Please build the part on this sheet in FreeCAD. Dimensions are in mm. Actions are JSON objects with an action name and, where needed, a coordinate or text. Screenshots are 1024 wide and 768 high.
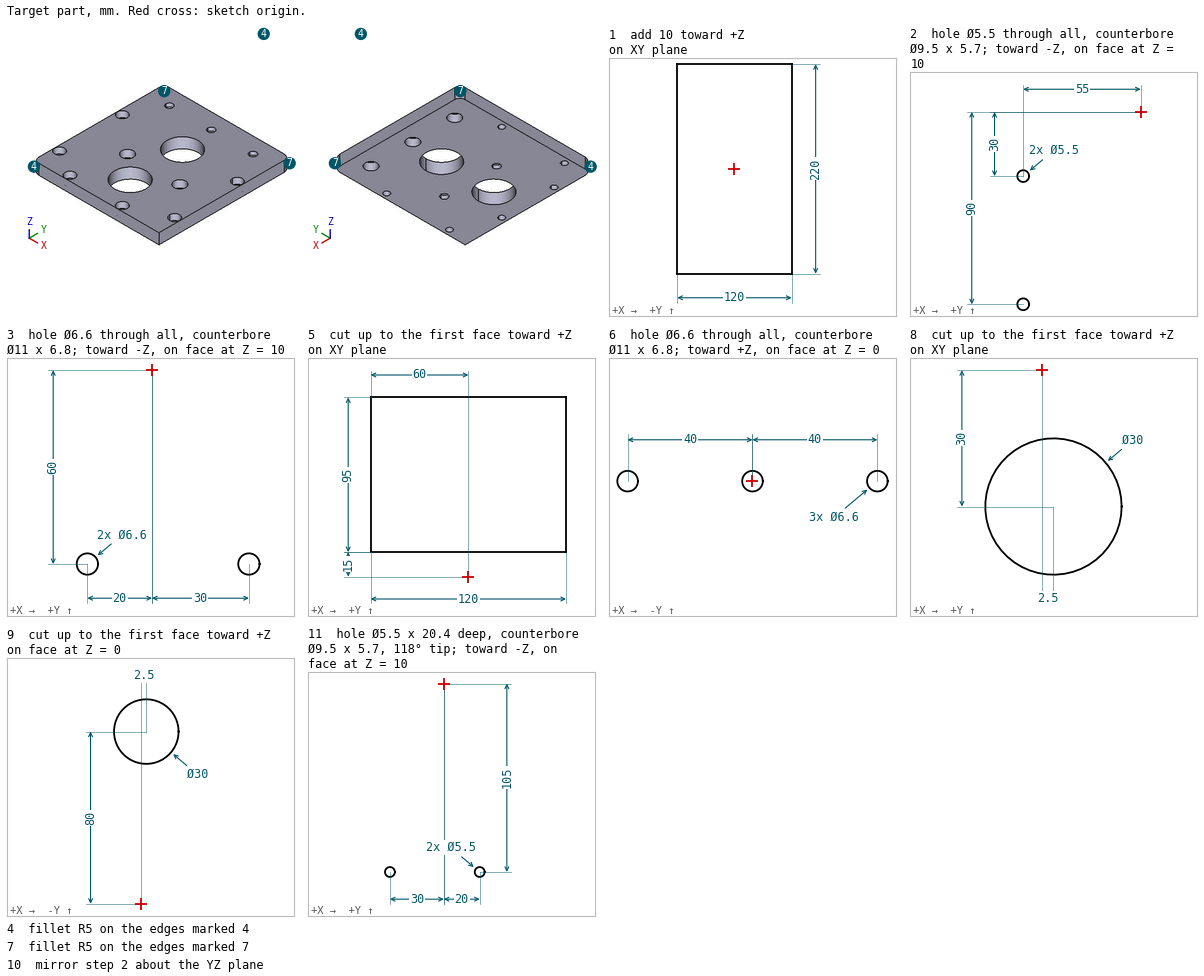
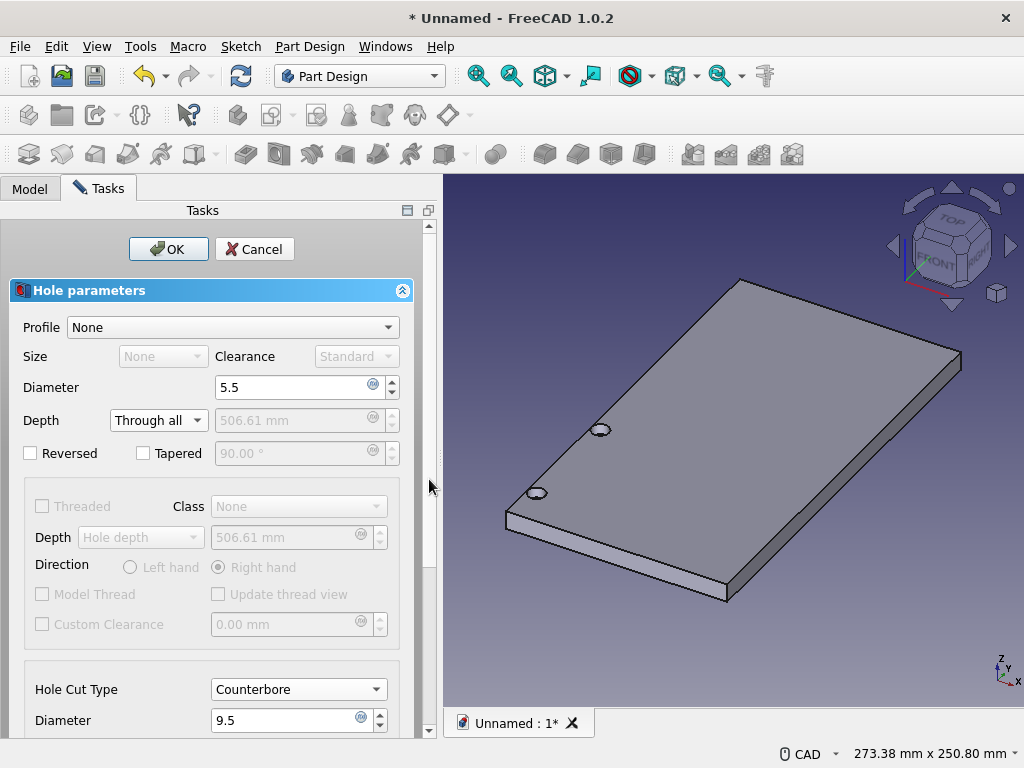
{"action": "left_click", "coordinate": [169, 249]}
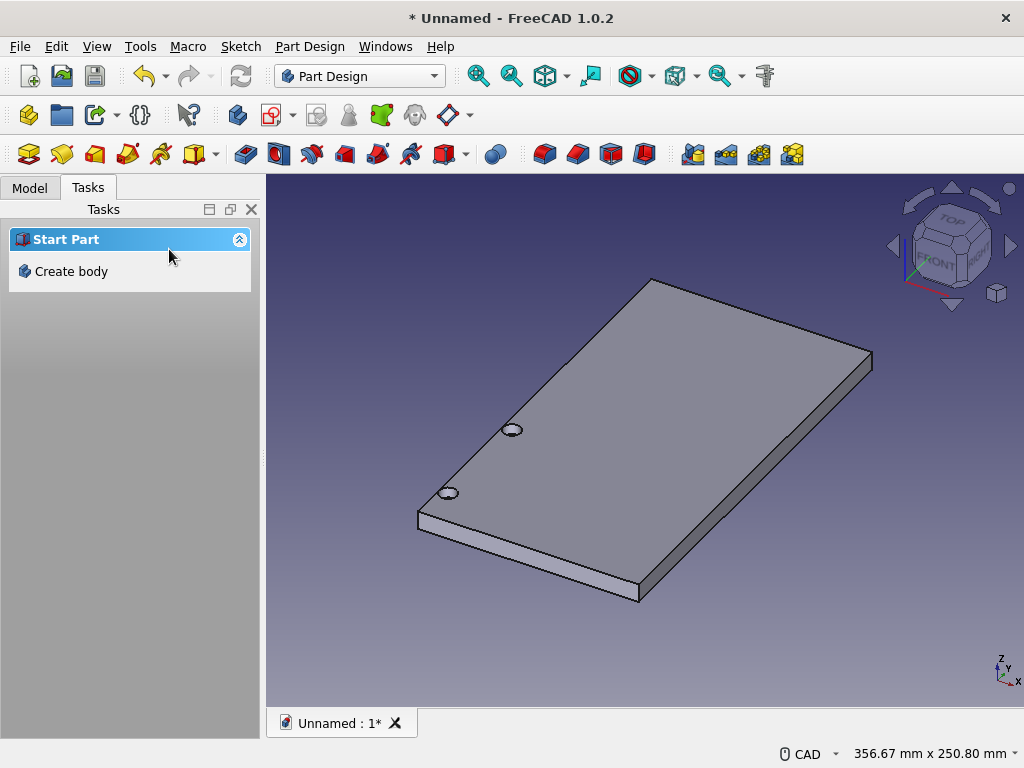
{"action": "left_click", "coordinate": [678, 398]}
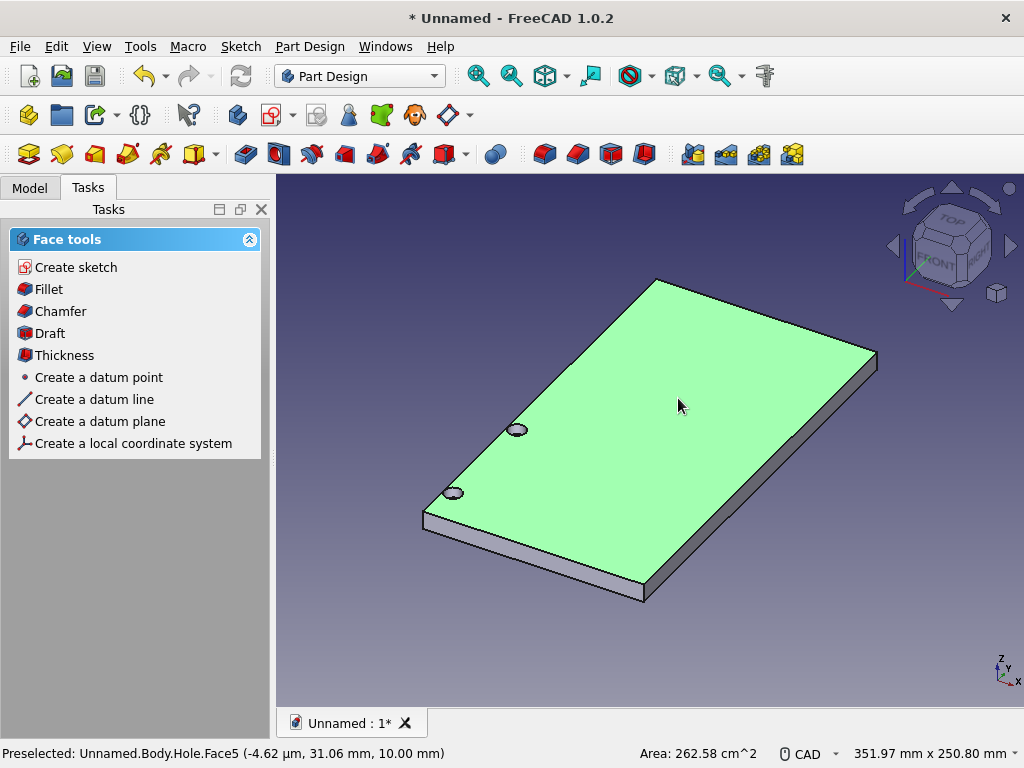
{"action": "left_click", "coordinate": [270, 116]}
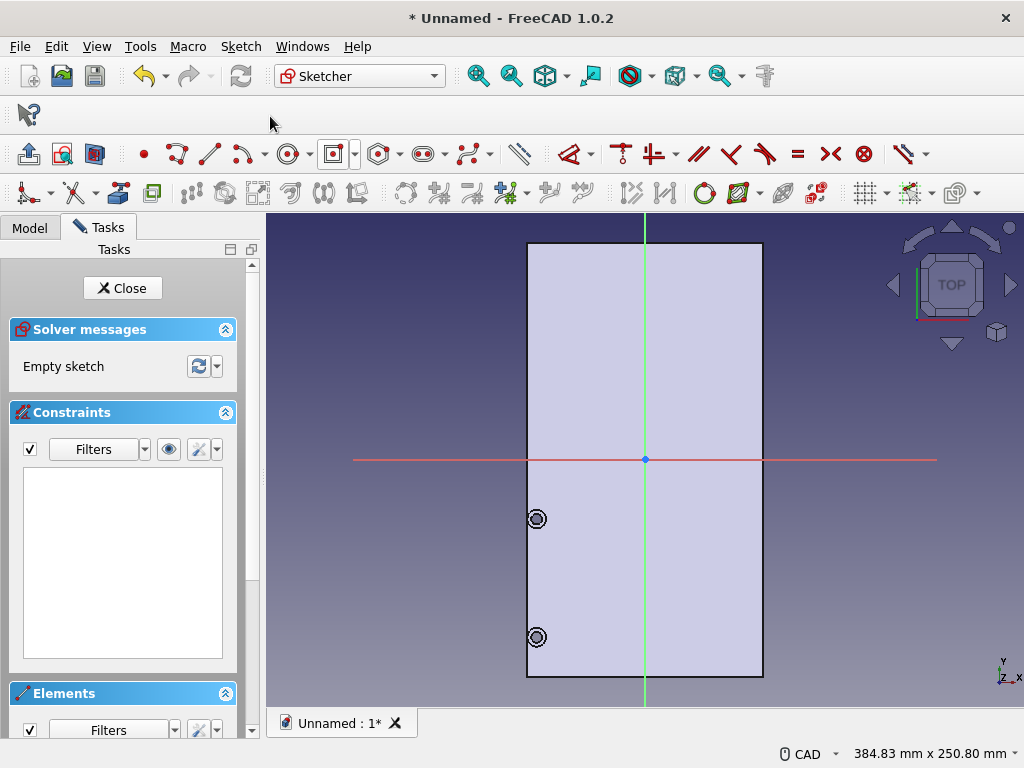
{"action": "scroll", "coordinate": [700, 559], "scroll_direction": "up", "scroll_amount": 5}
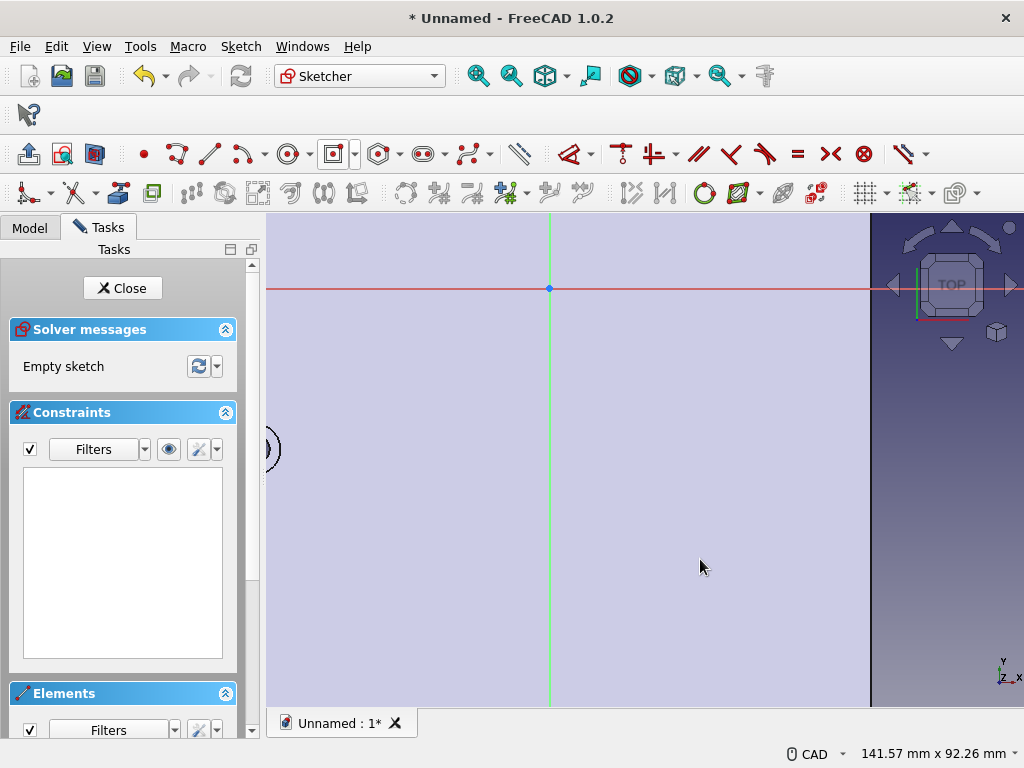
{"action": "left_click", "coordinate": [288, 154]}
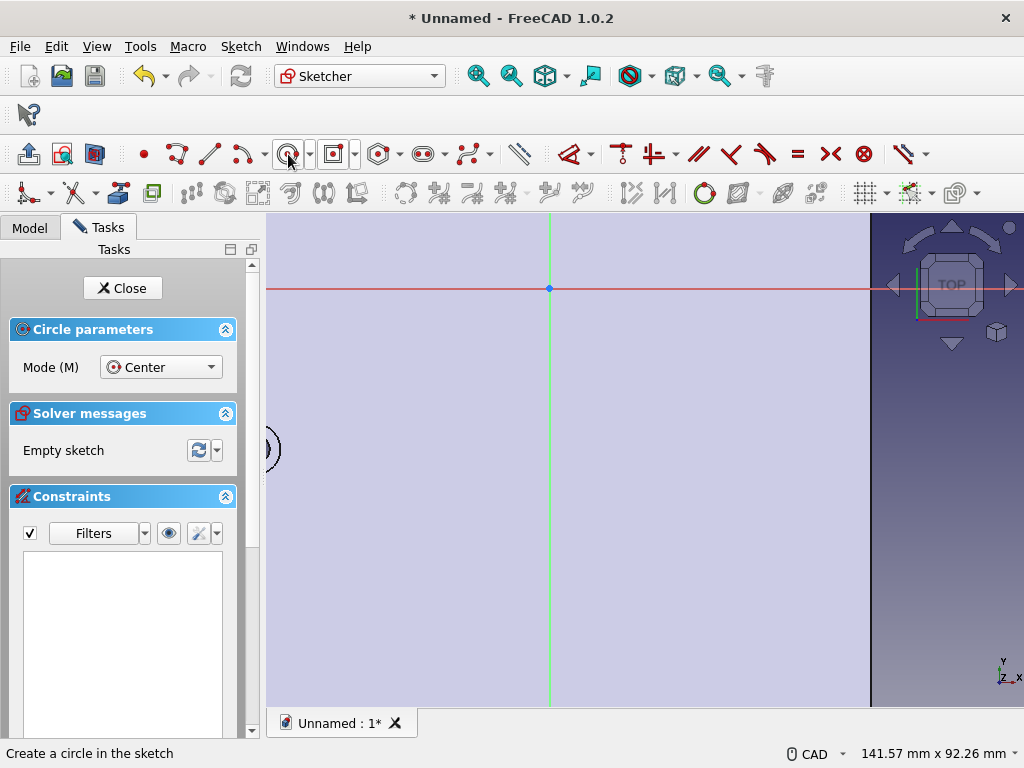
{"action": "scroll", "coordinate": [442, 610], "scroll_direction": "up", "scroll_amount": 2}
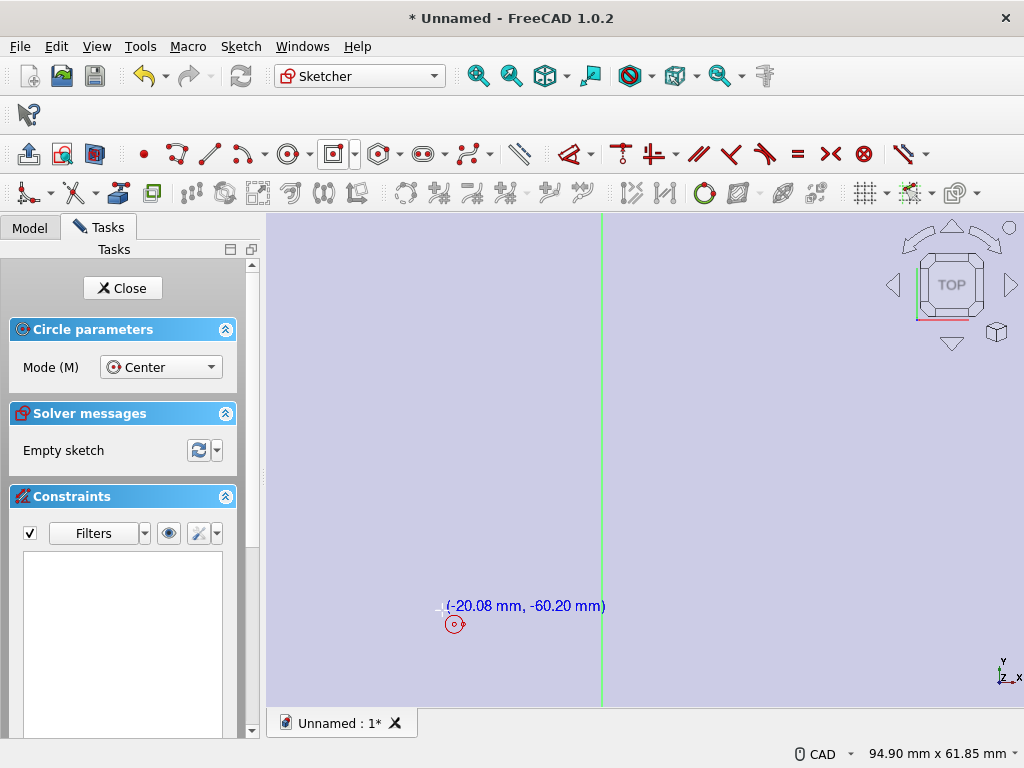
{"action": "left_click", "coordinate": [443, 610]}
{"action": "left_click", "coordinate": [461, 591]}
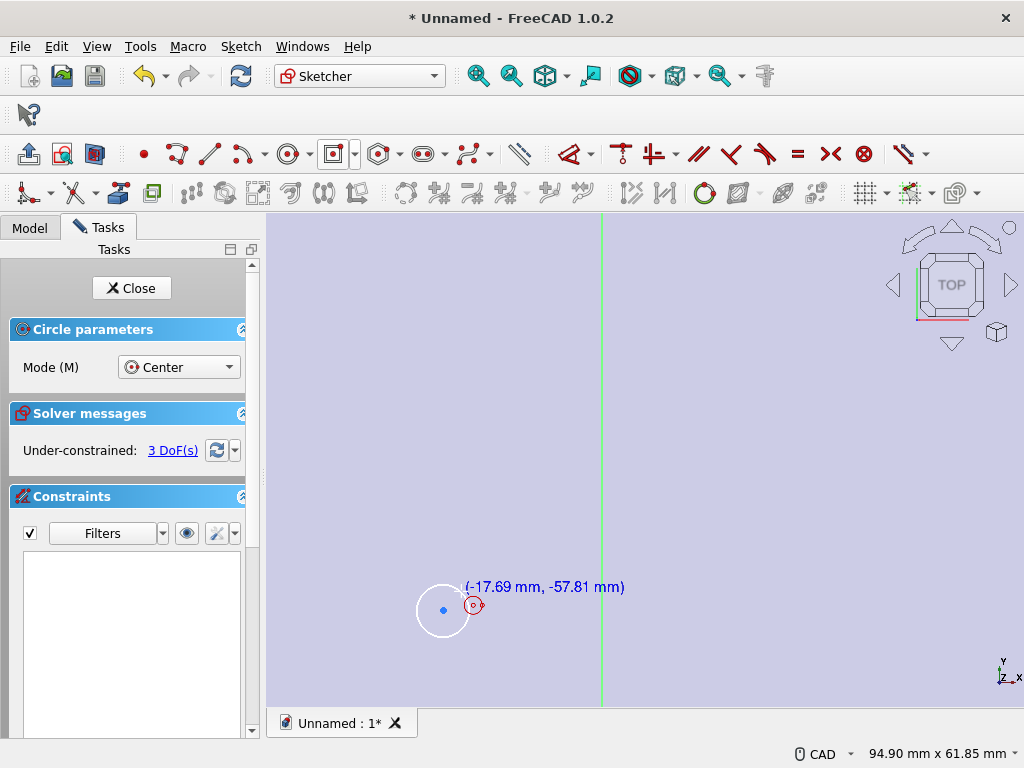
{"action": "left_click", "coordinate": [842, 610]}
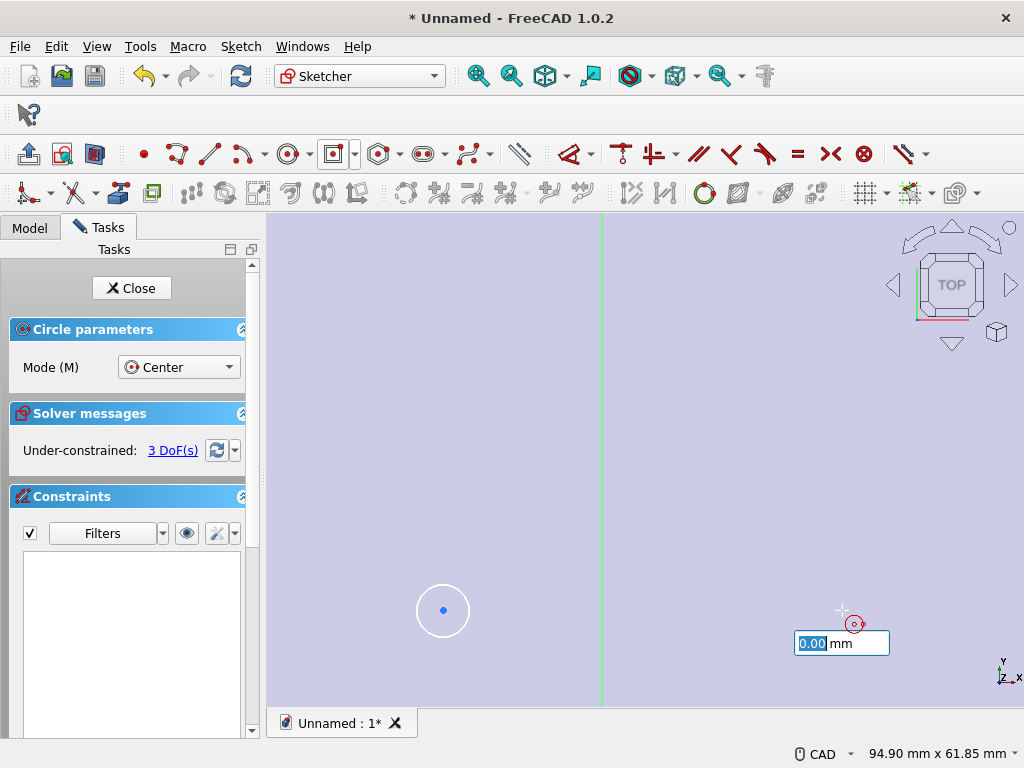
{"action": "scroll", "coordinate": [443, 616], "scroll_direction": "down", "scroll_amount": 2}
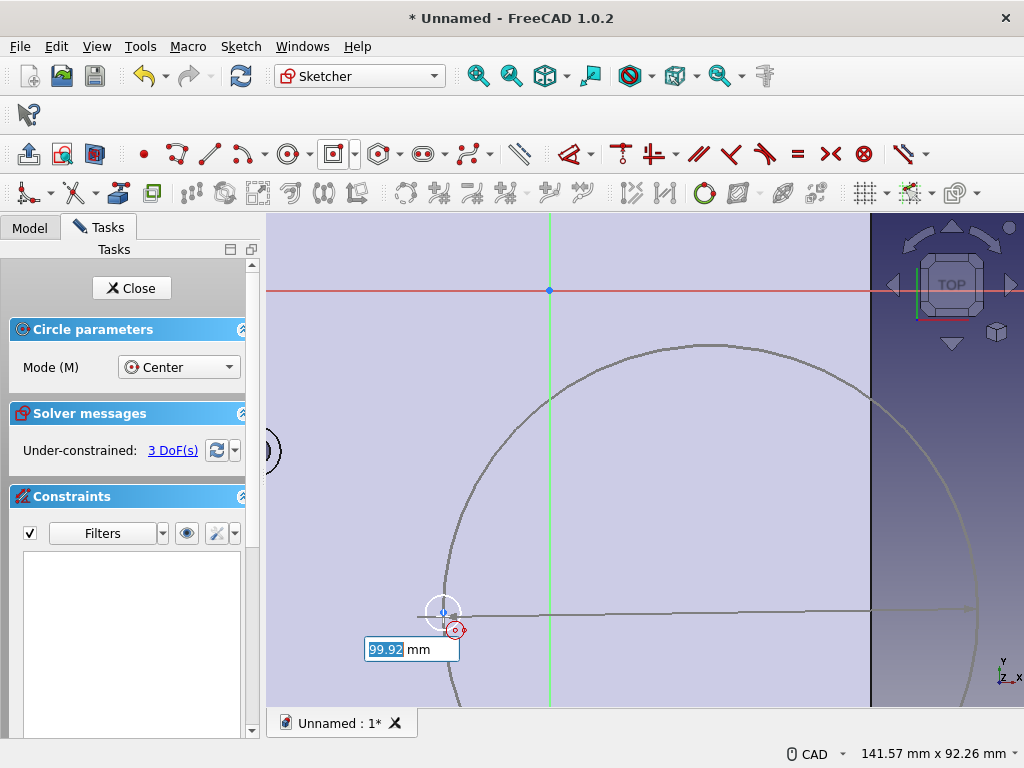
{"action": "left_click", "coordinate": [723, 599]}
{"action": "key", "text": "Escape"}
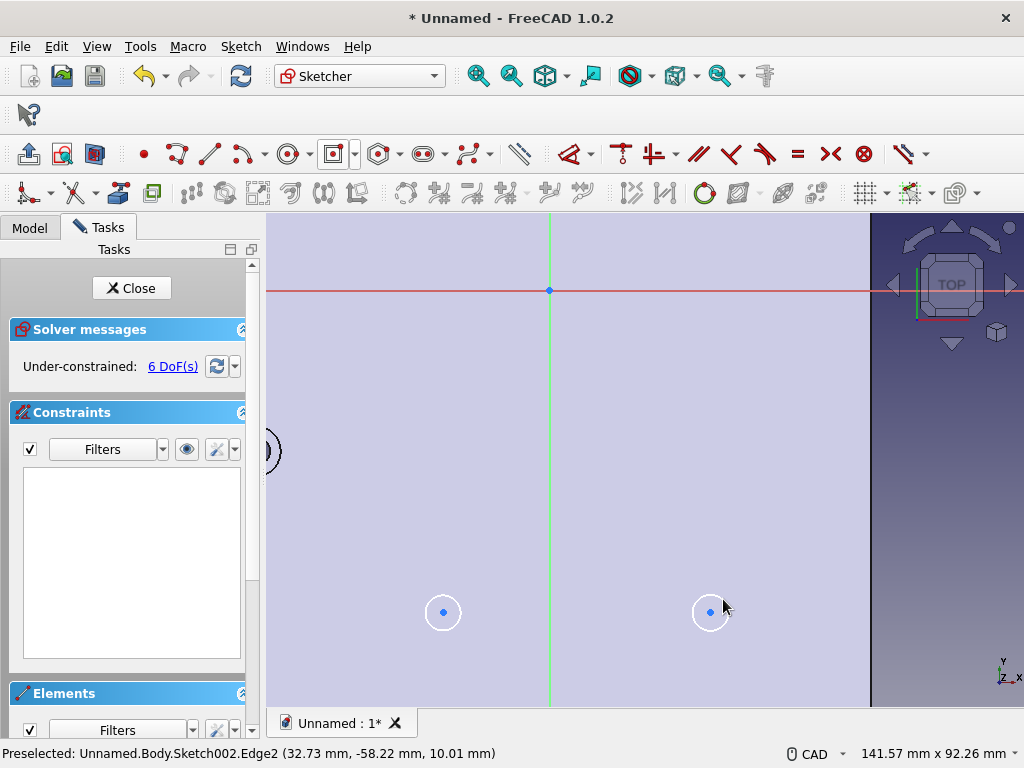
{"action": "left_click", "coordinate": [455, 600]}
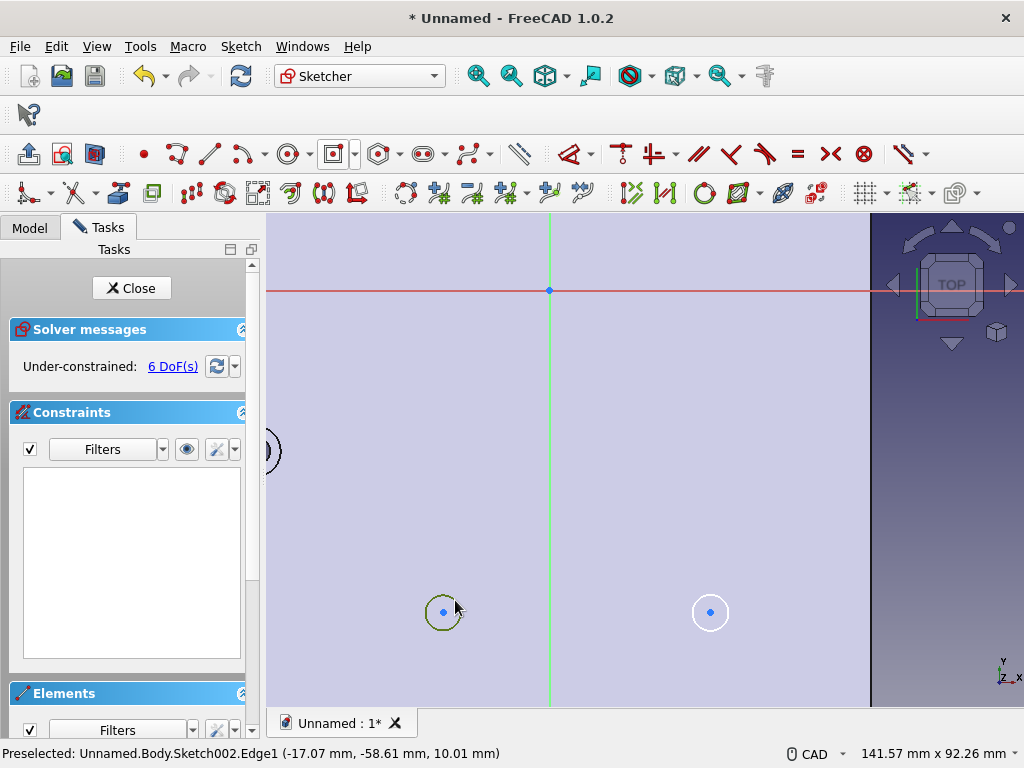
{"action": "left_click", "coordinate": [723, 600]}